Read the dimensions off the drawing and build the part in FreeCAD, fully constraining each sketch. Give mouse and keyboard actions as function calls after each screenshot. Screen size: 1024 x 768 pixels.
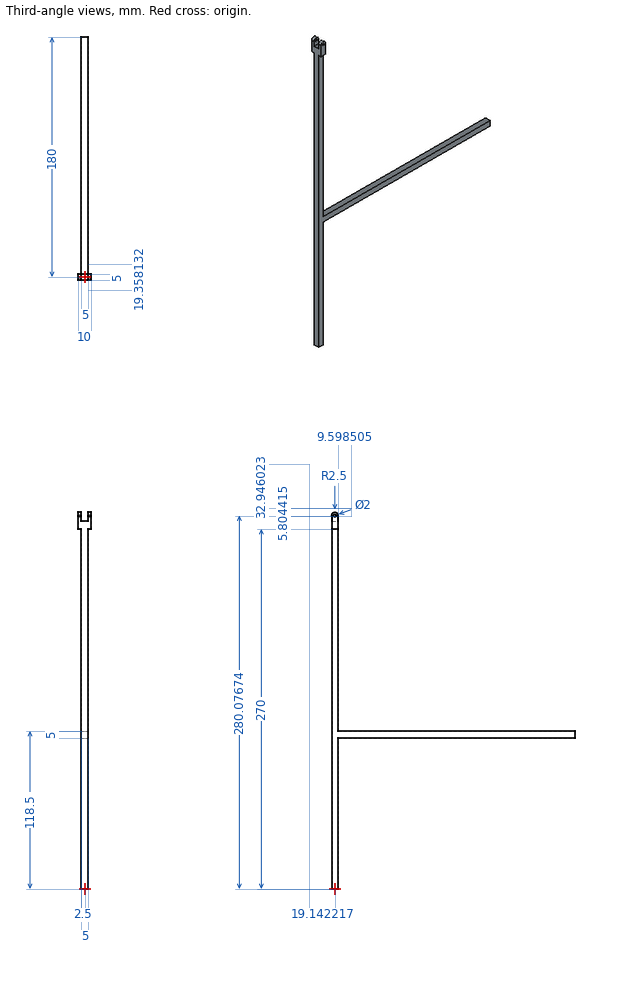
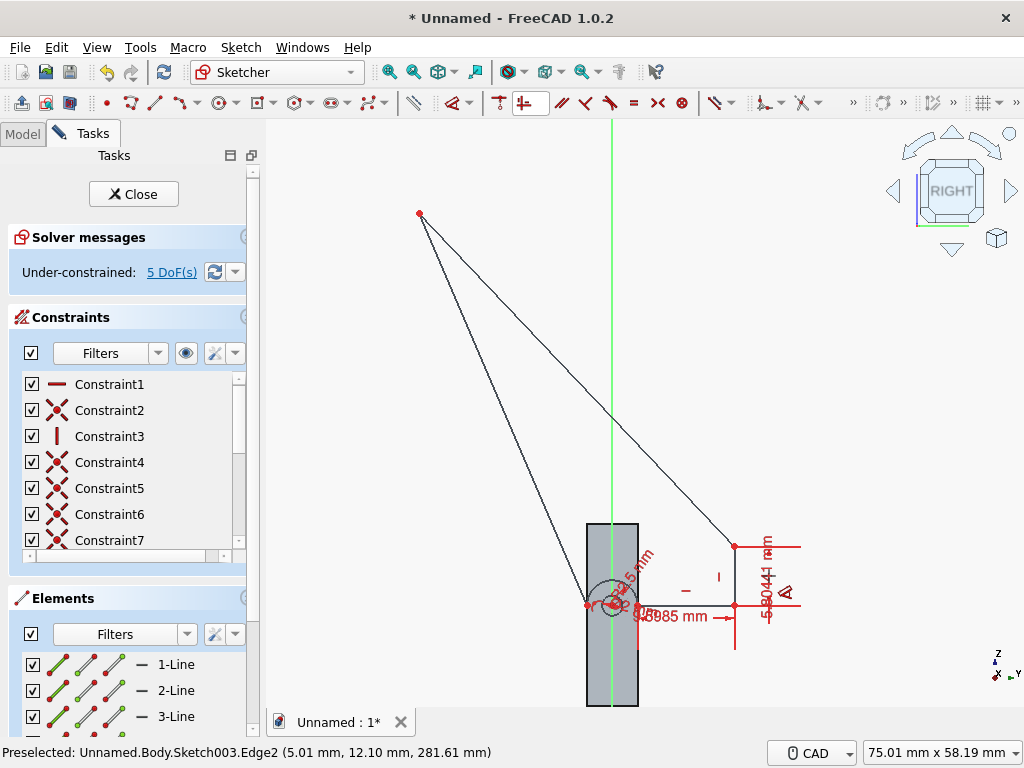
click(612, 606)
click(646, 642)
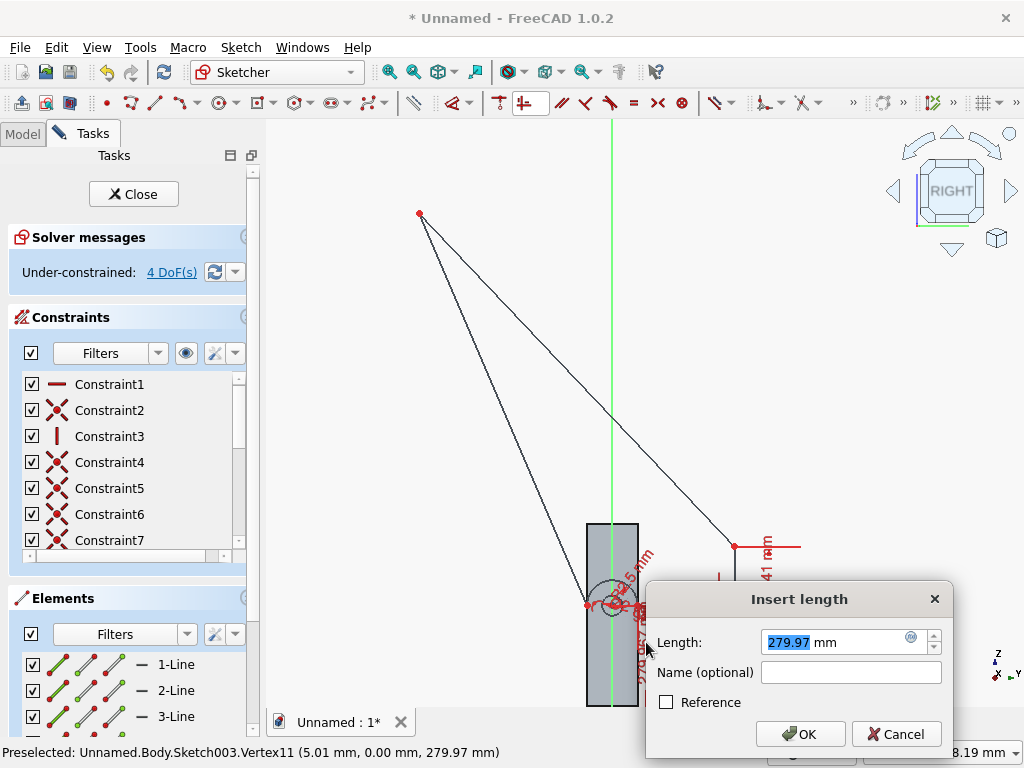
text(280.07674)
key(Return)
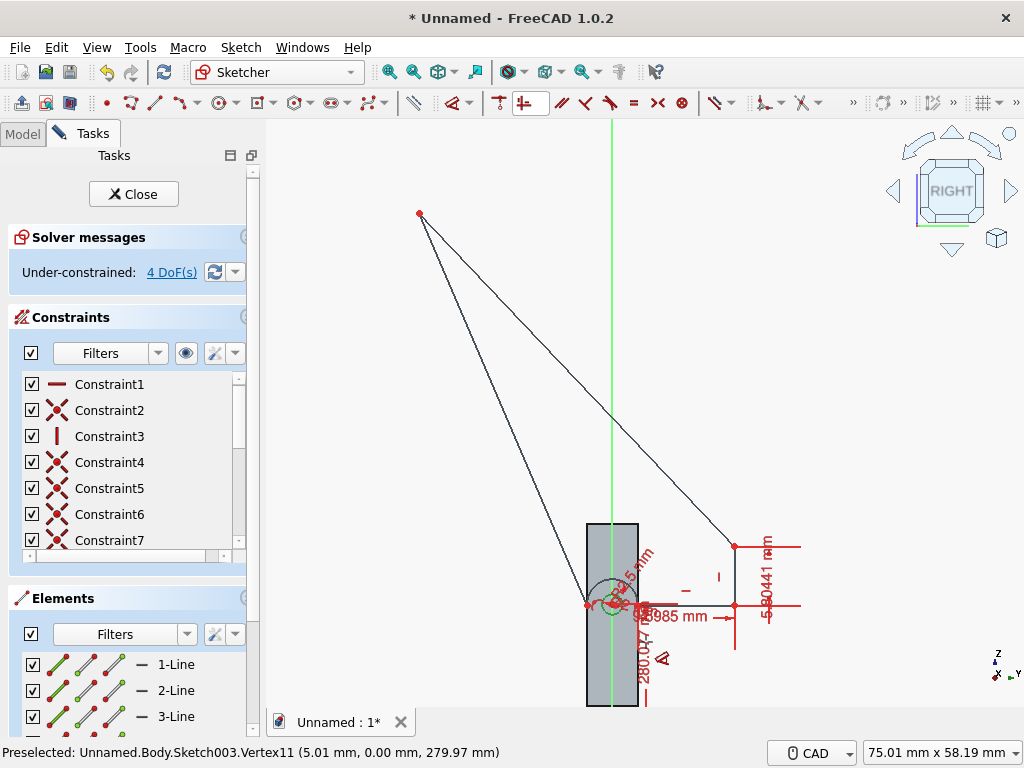
click(638, 606)
click(672, 668)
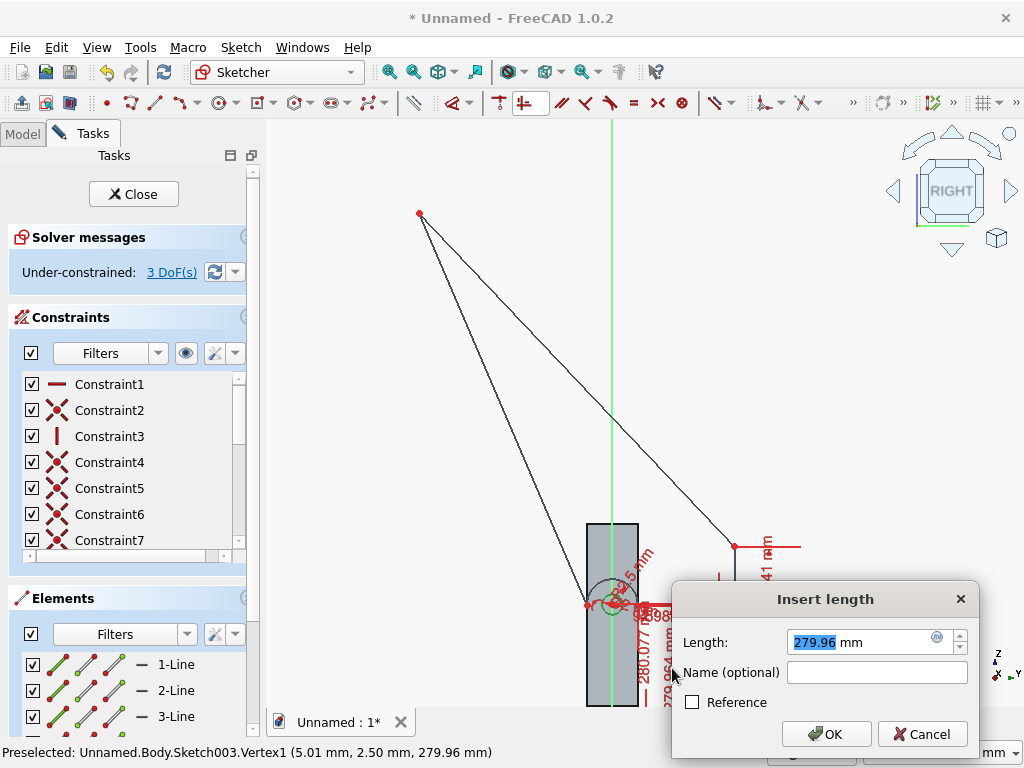
text(280.07674)
key(Return)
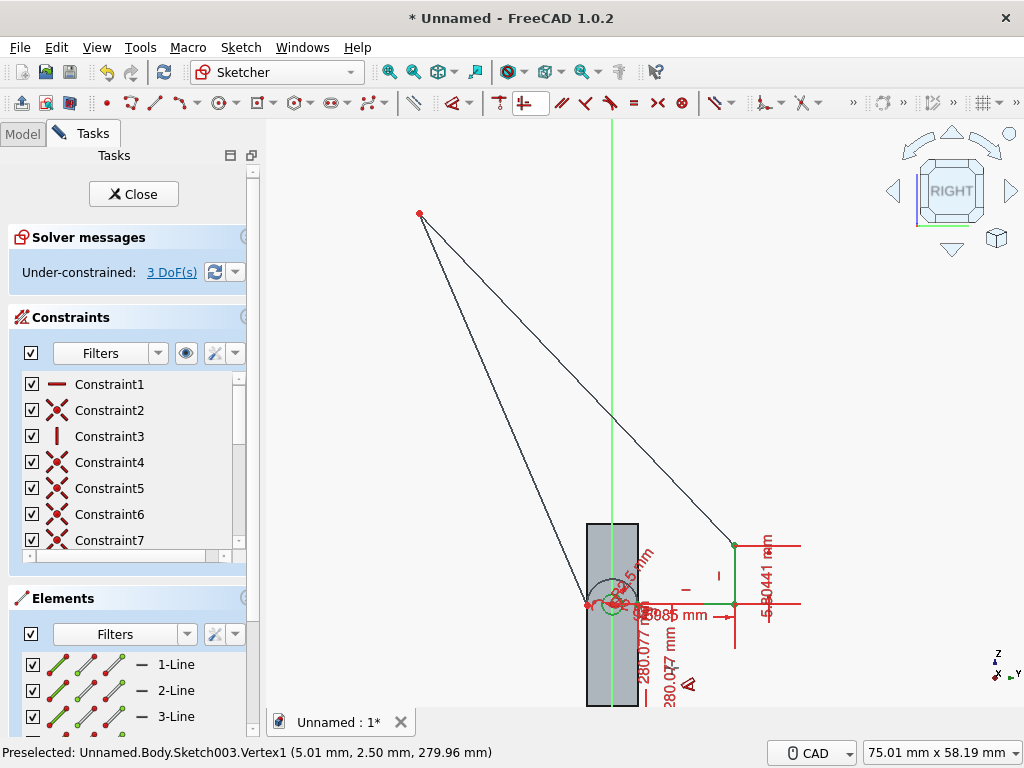
click(419, 214)
click(516, 180)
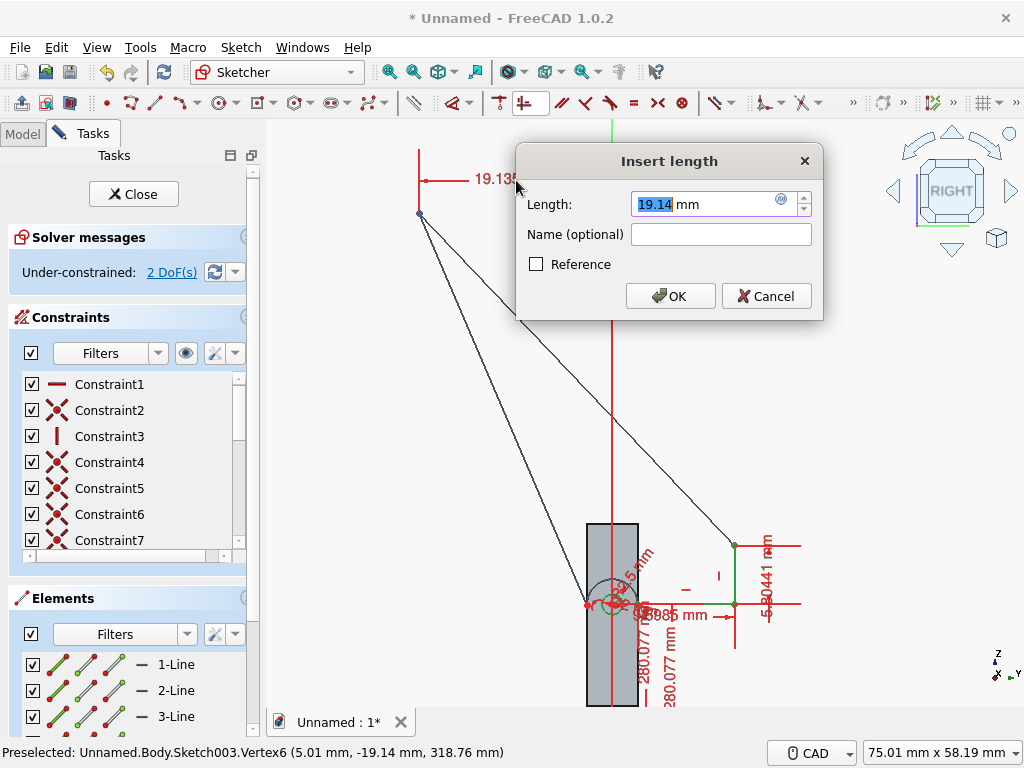
text(19.142217)
key(Return)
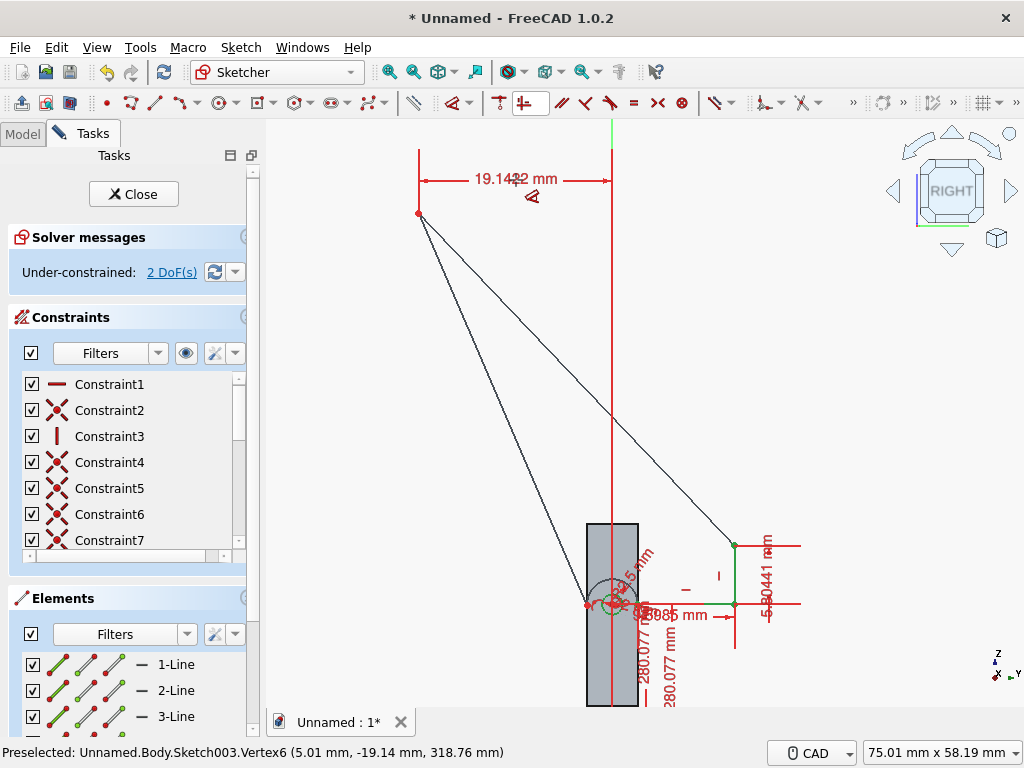
click(587, 606)
click(553, 642)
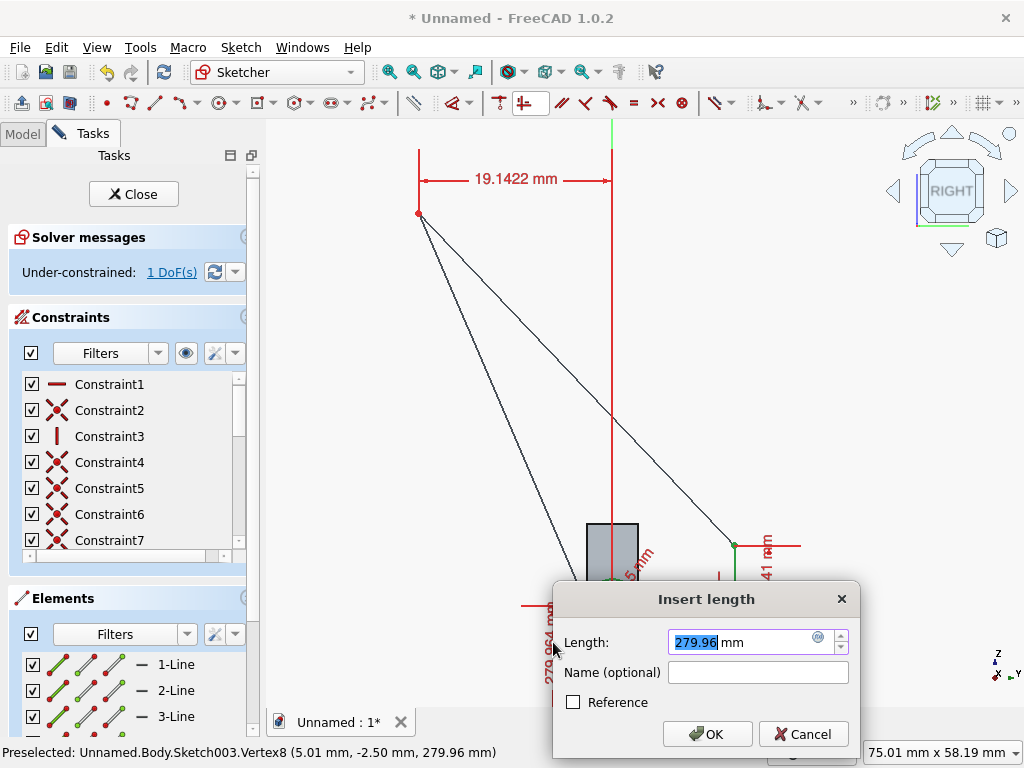
text(280.07674)
key(Return)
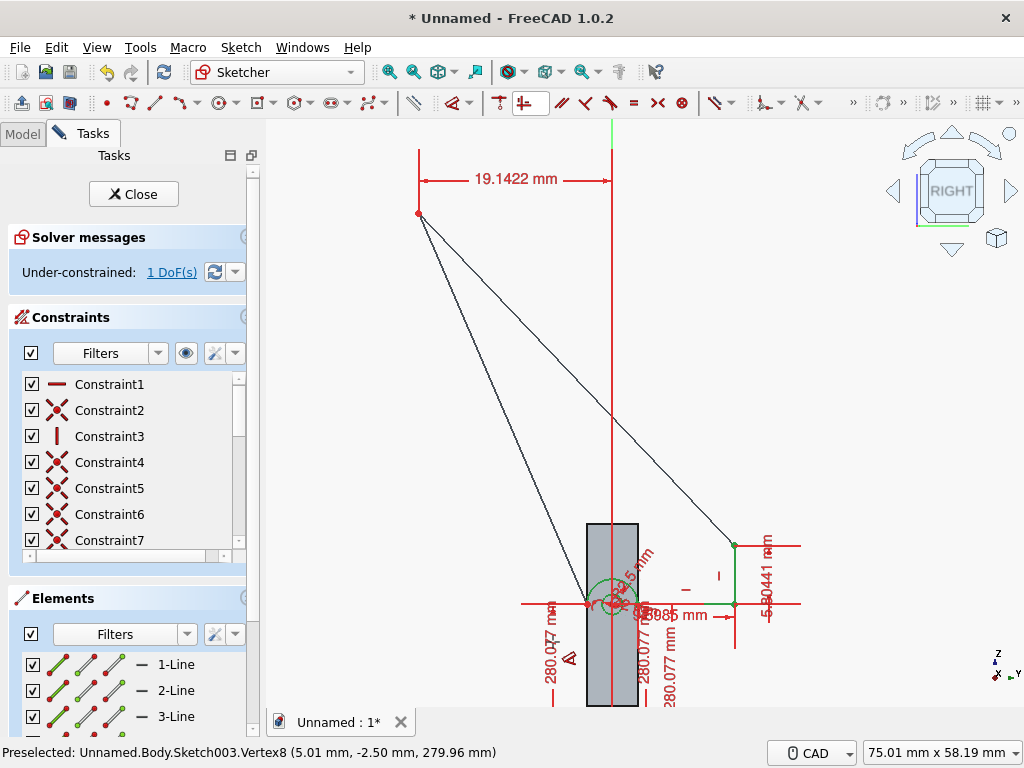
click(640, 446)
click(769, 380)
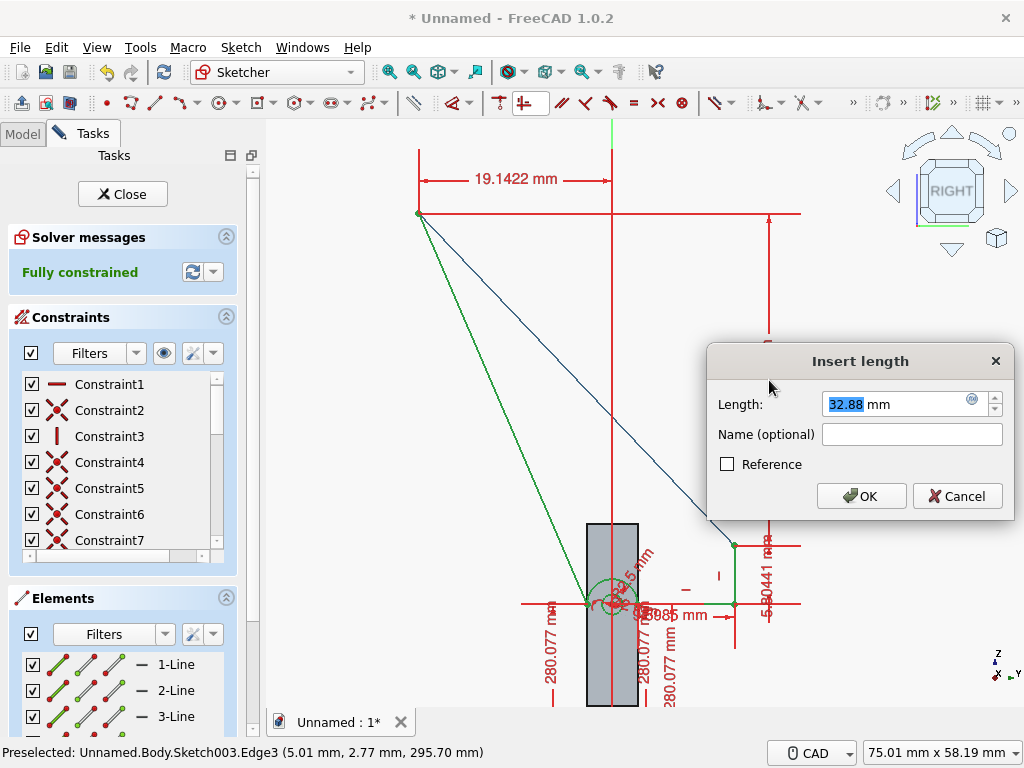
text(32.946023)
key(Return)
key(Escape)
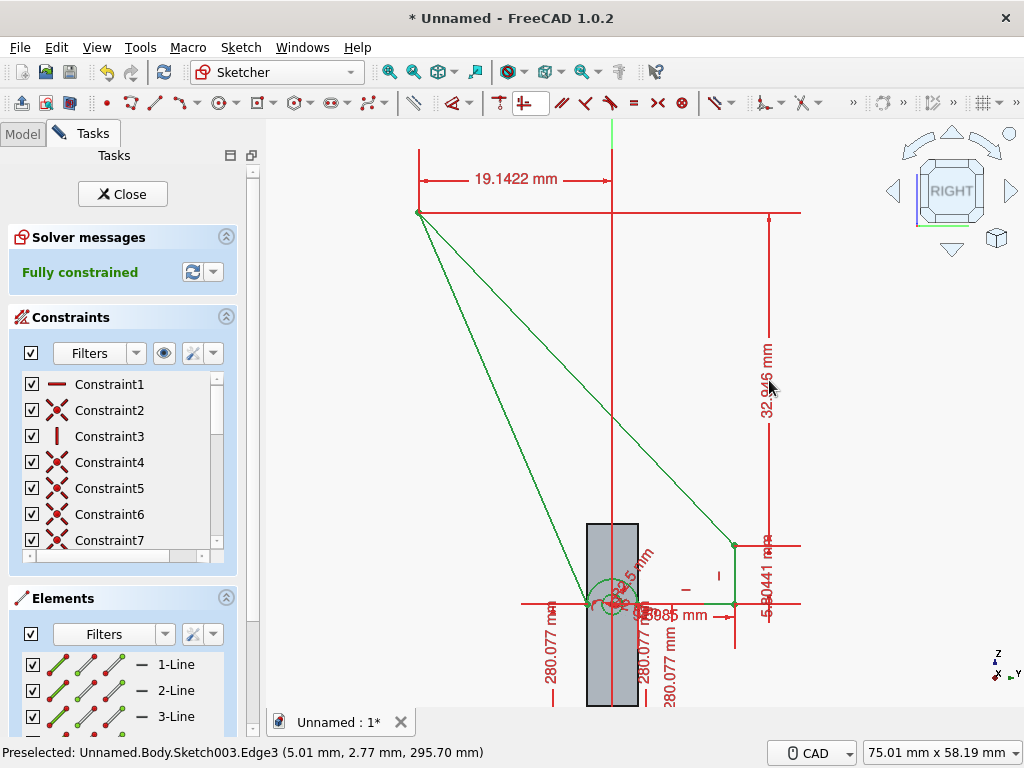
click(123, 194)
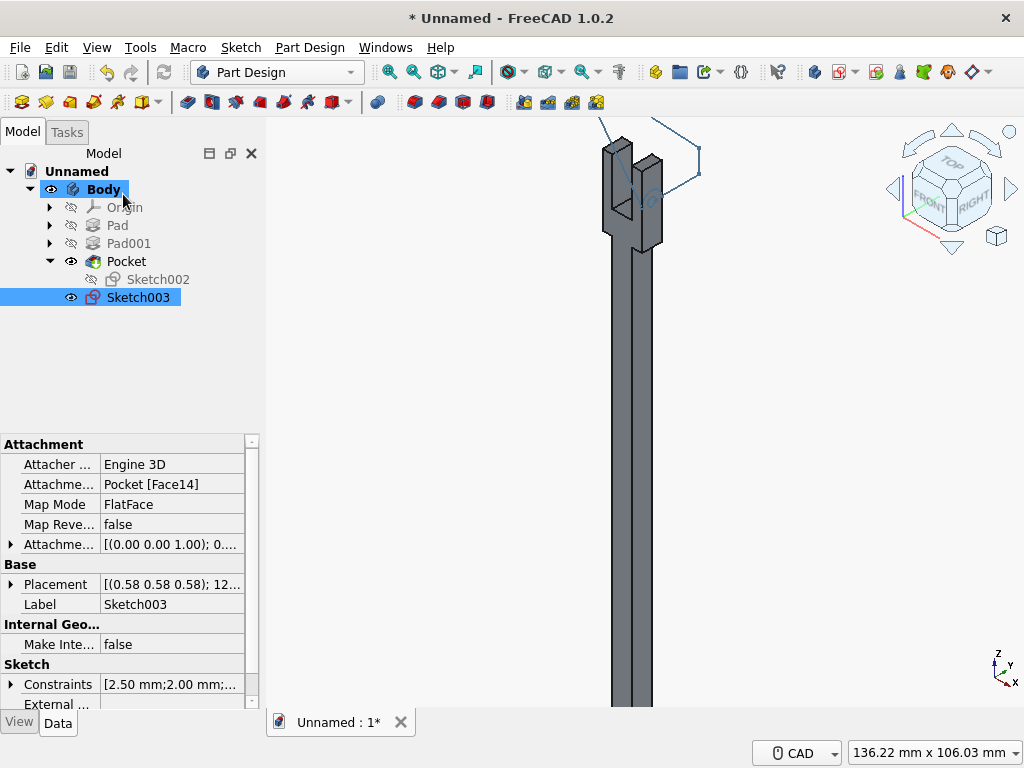
click(188, 102)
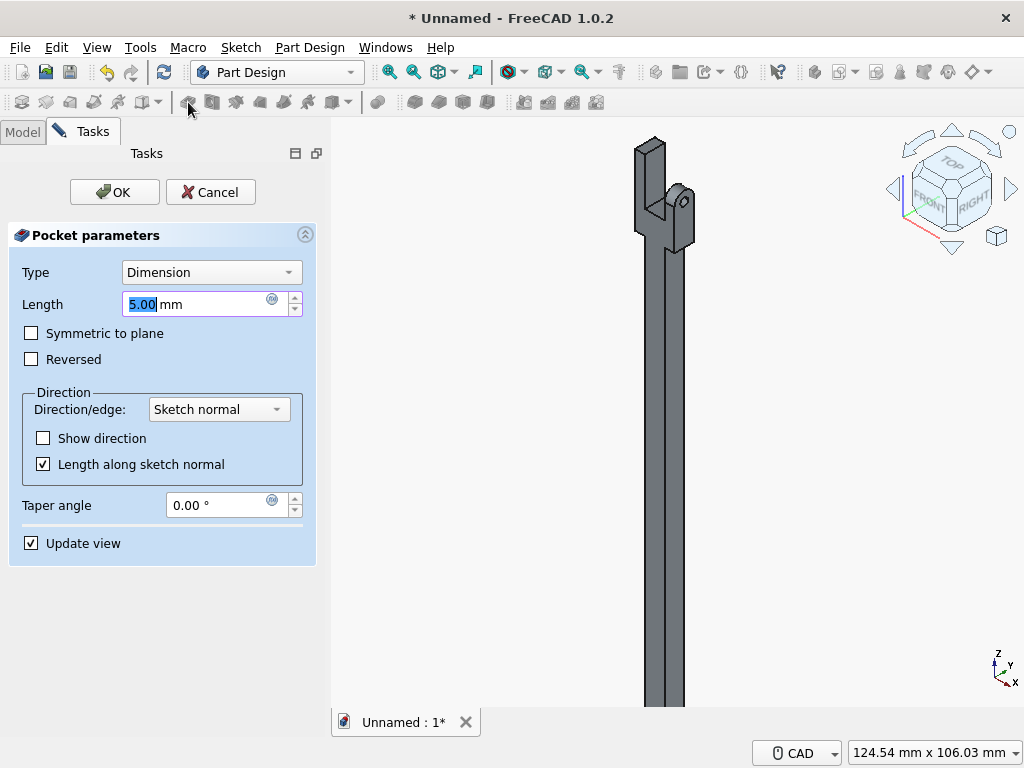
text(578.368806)
key(Tab)